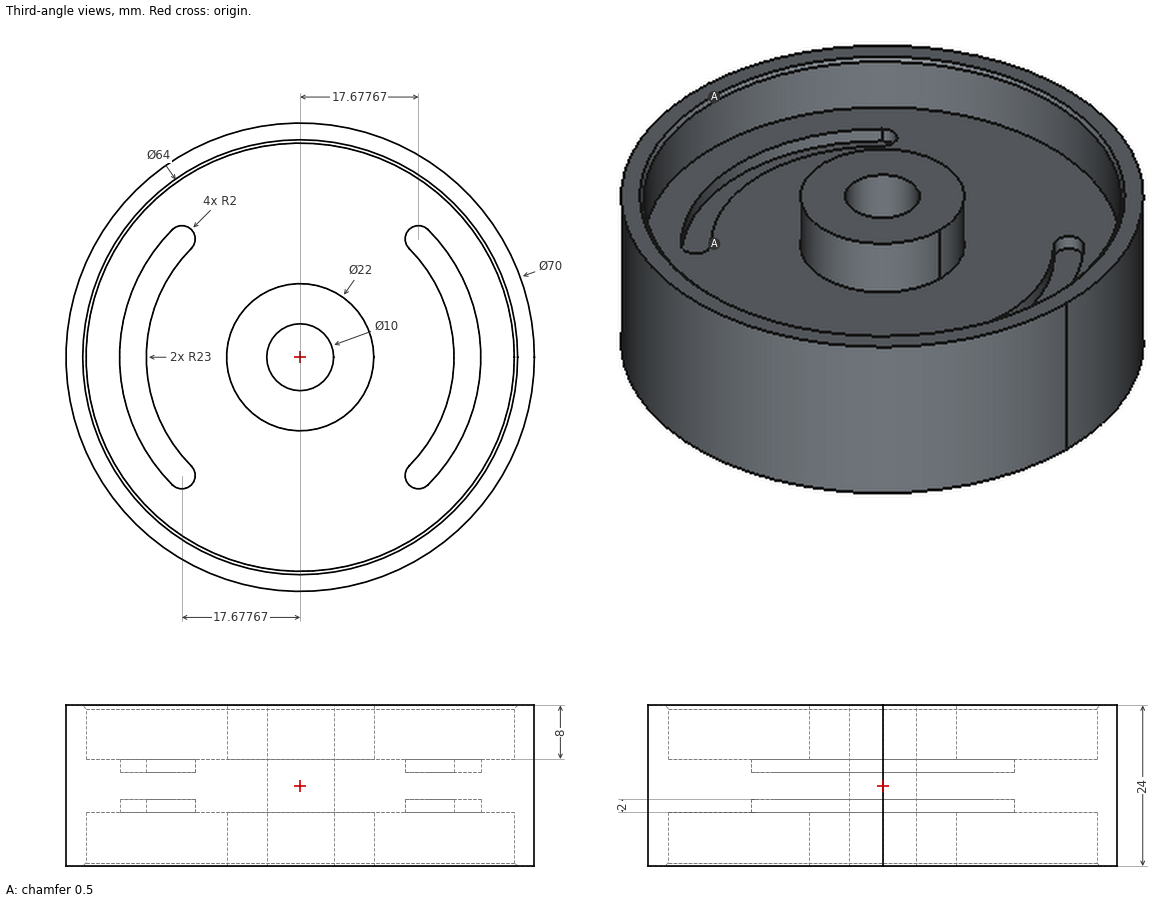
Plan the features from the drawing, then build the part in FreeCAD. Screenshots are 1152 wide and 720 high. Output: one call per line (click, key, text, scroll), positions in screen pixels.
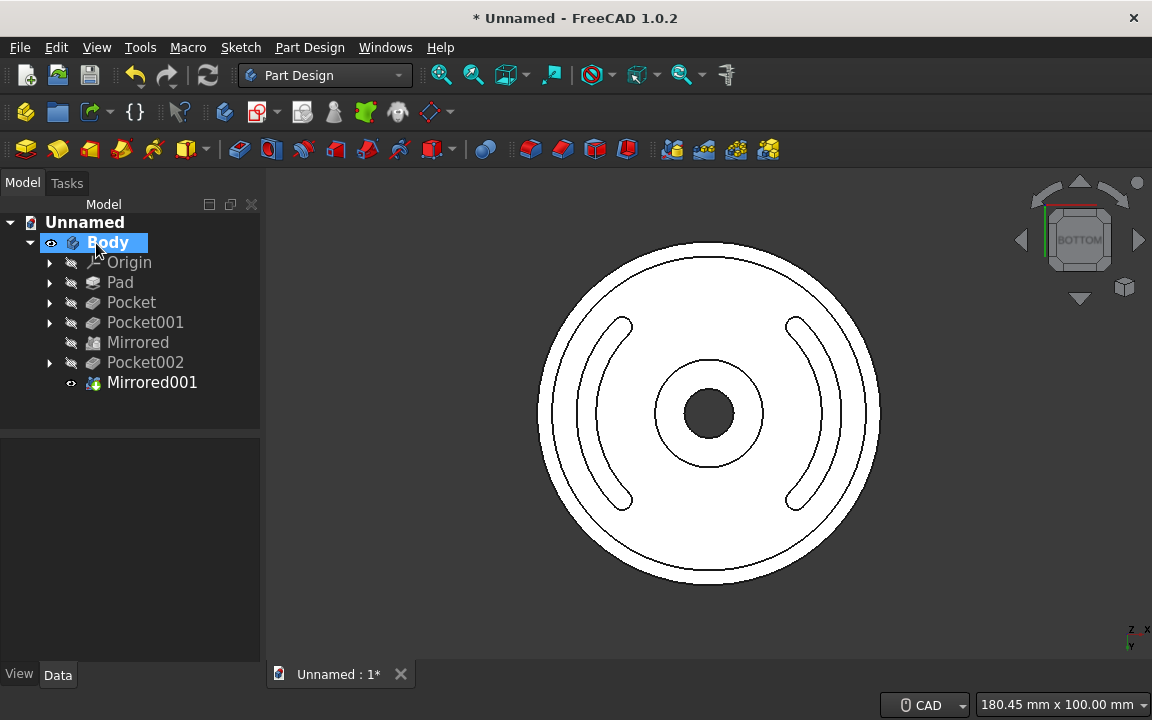
click(582, 320)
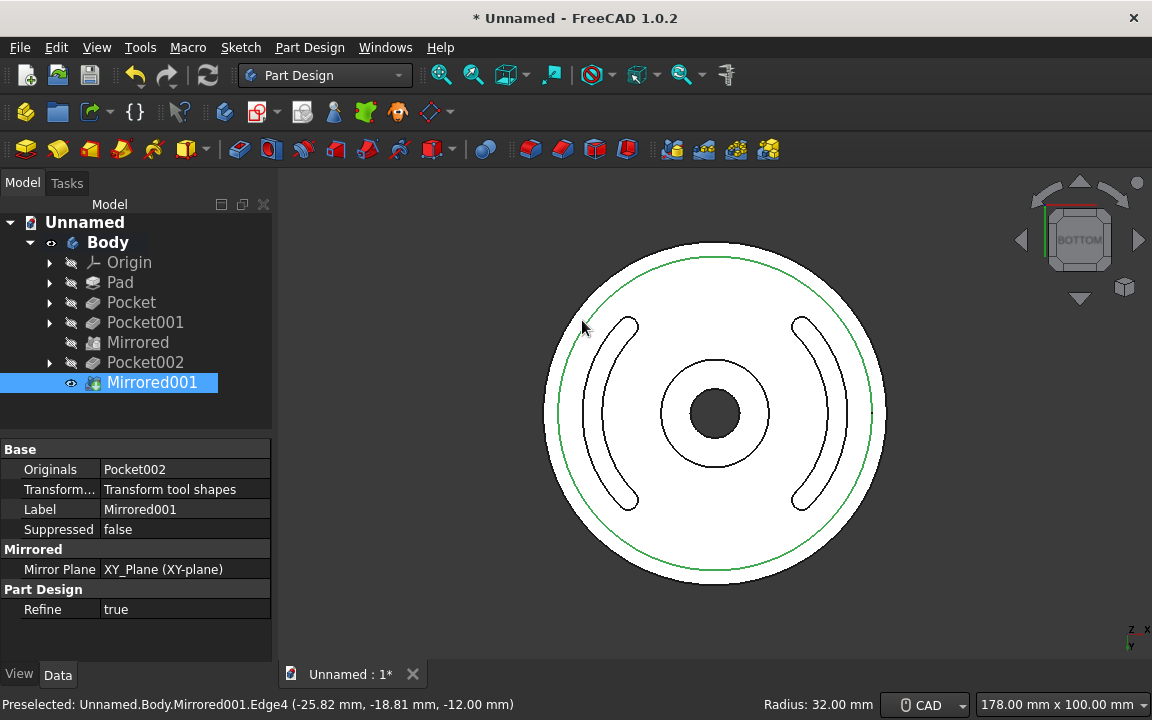
key(0)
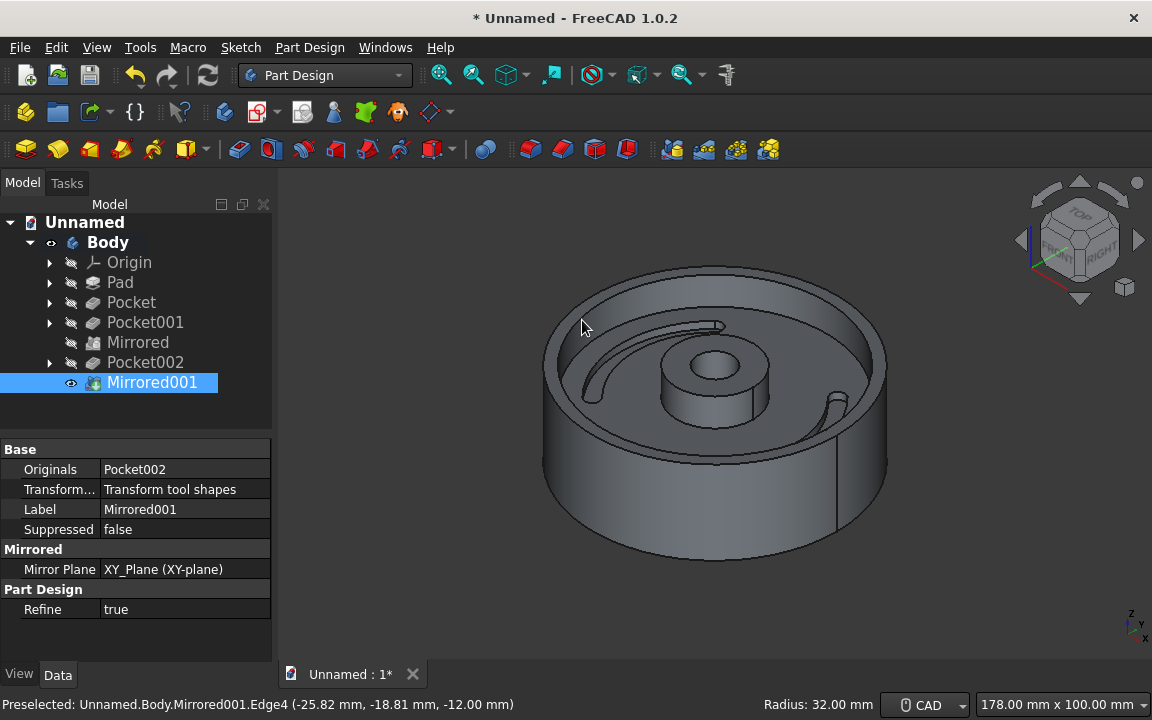
click(604, 300, ctrl)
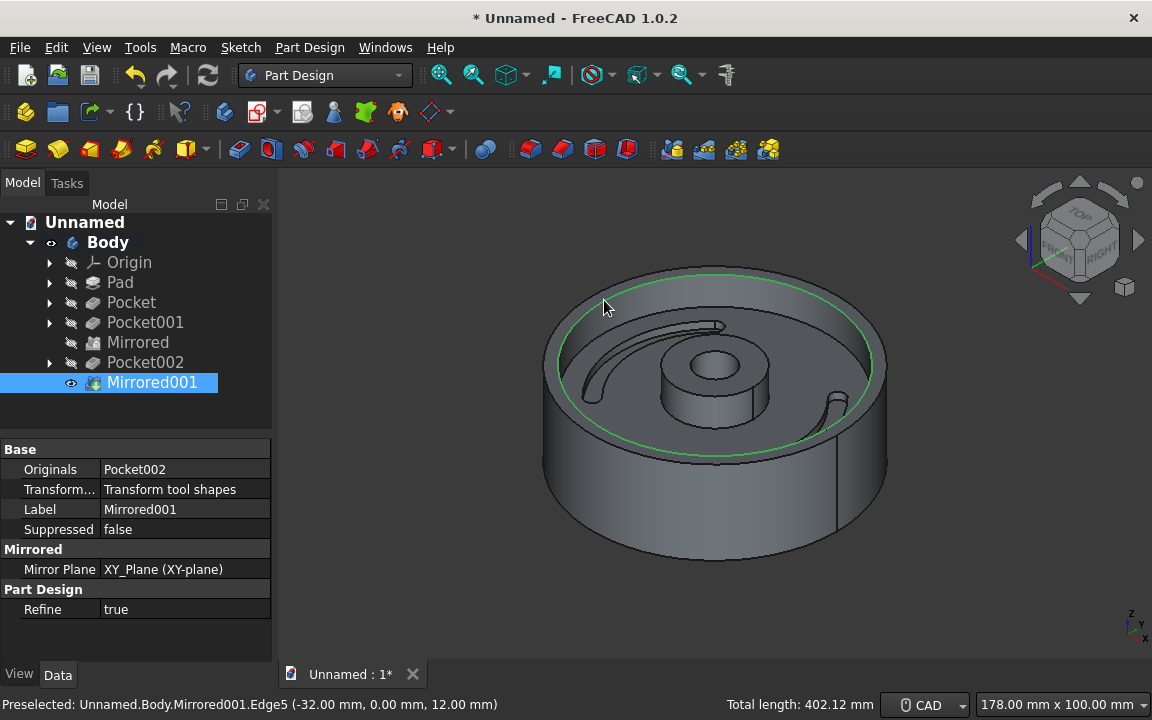
click(564, 150)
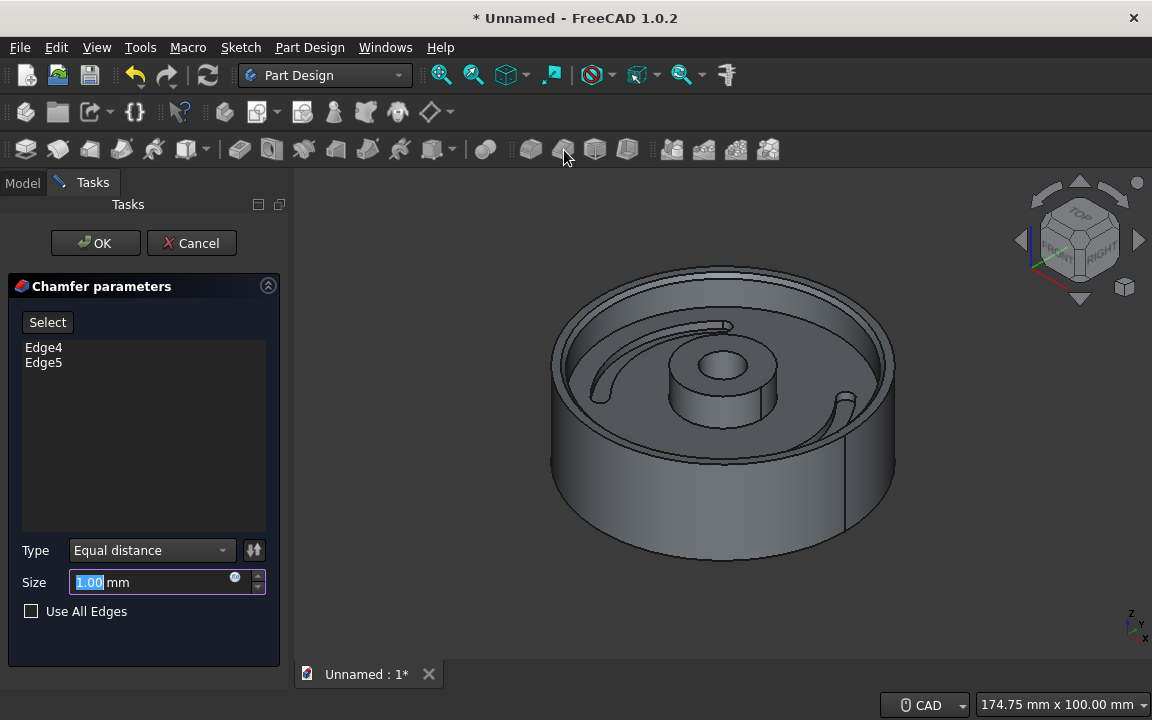
text(0.5)
key(Tab)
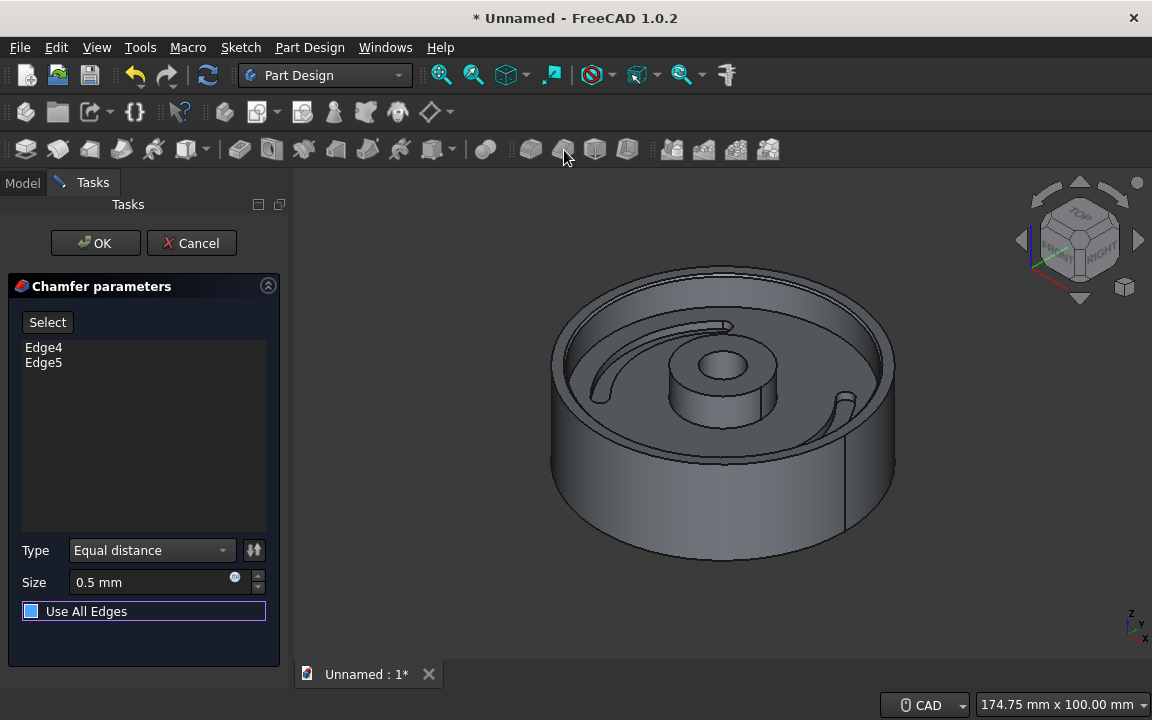
click(96, 243)